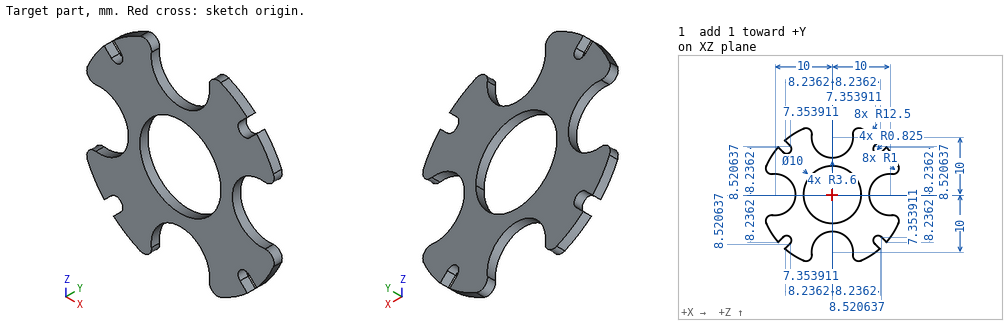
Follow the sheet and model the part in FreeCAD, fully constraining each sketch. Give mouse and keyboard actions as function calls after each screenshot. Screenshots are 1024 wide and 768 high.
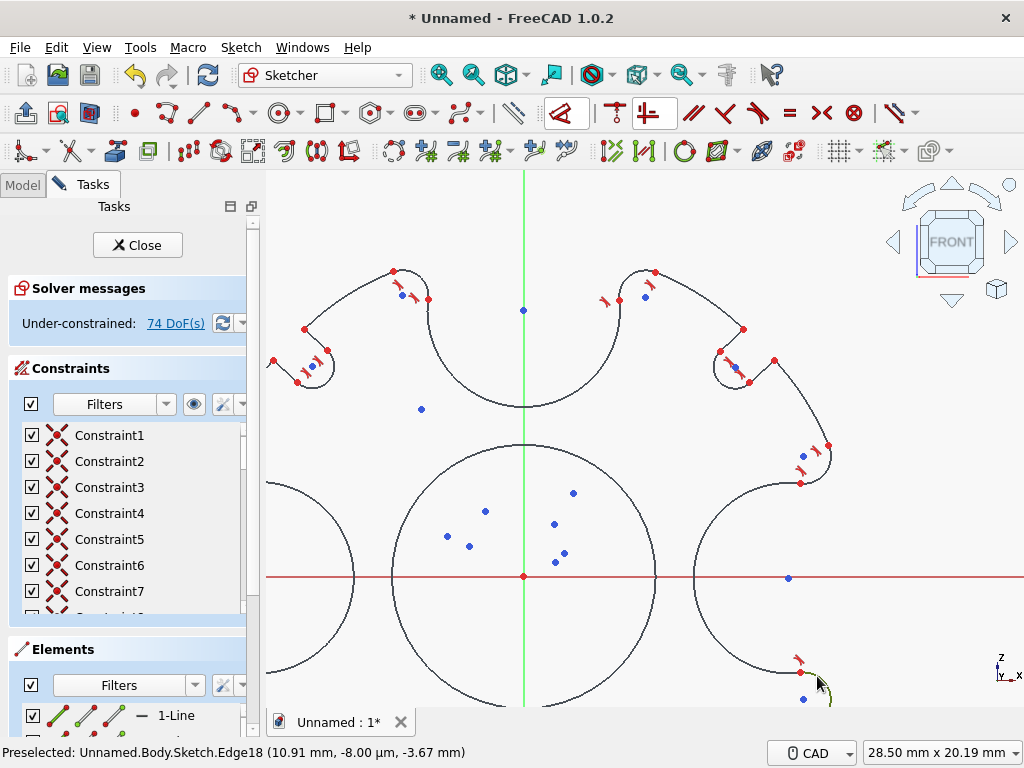
scroll(641, 270, down, 3)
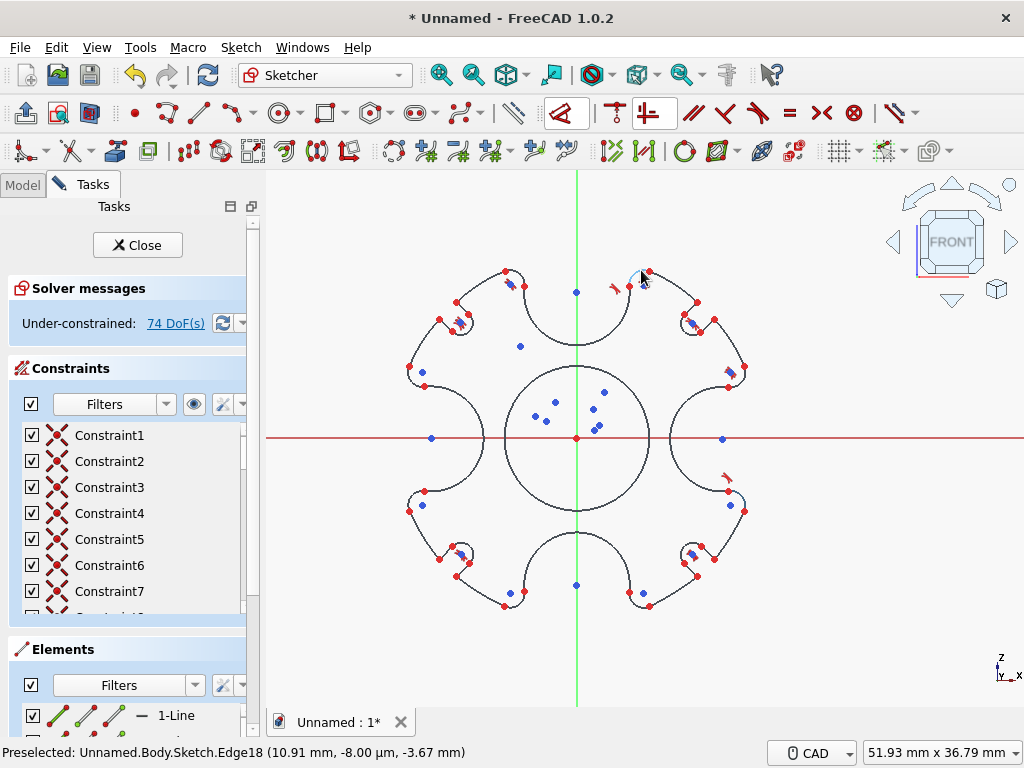
click(725, 546)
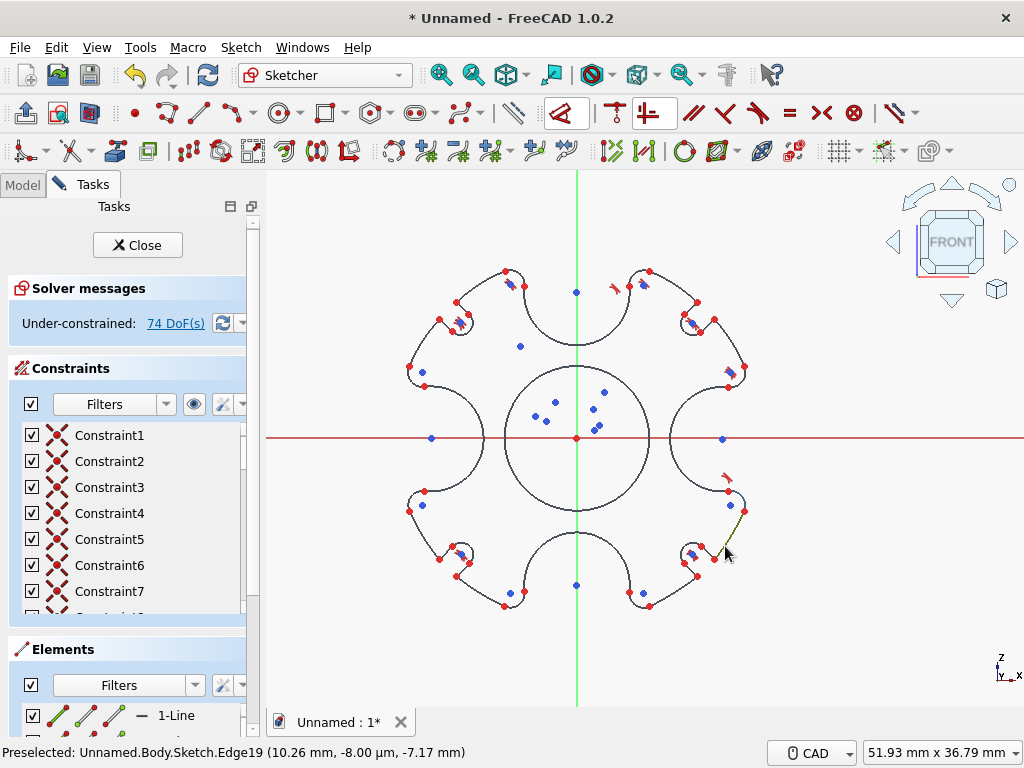
click(758, 114)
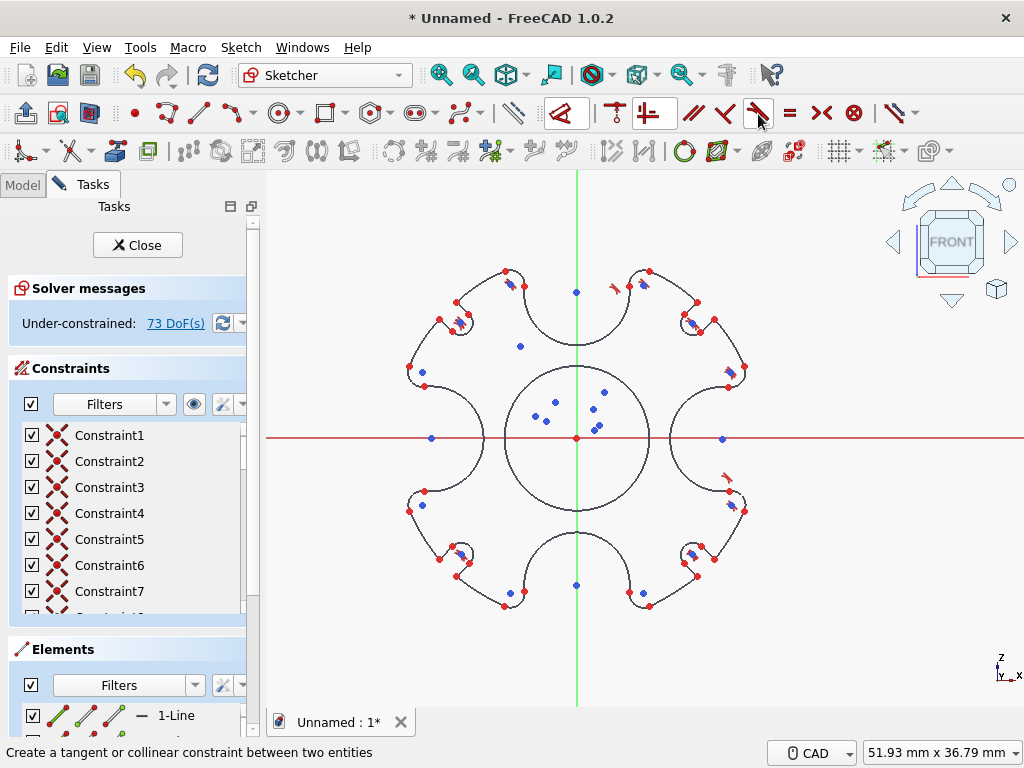
click(665, 599)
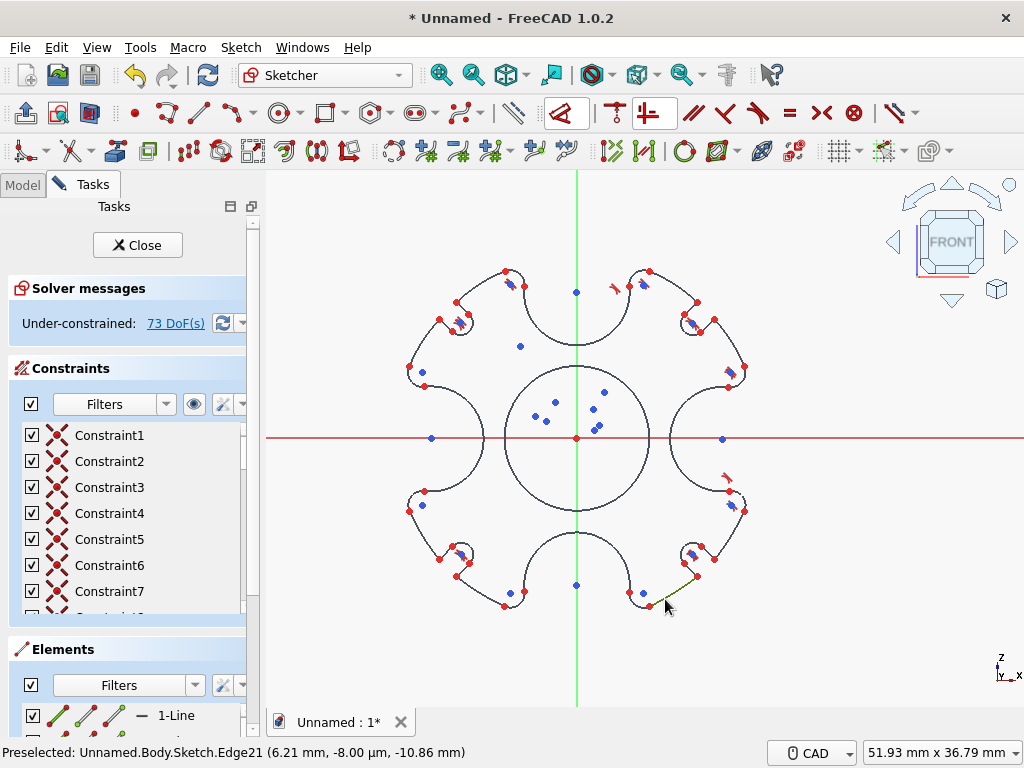
click(635, 605)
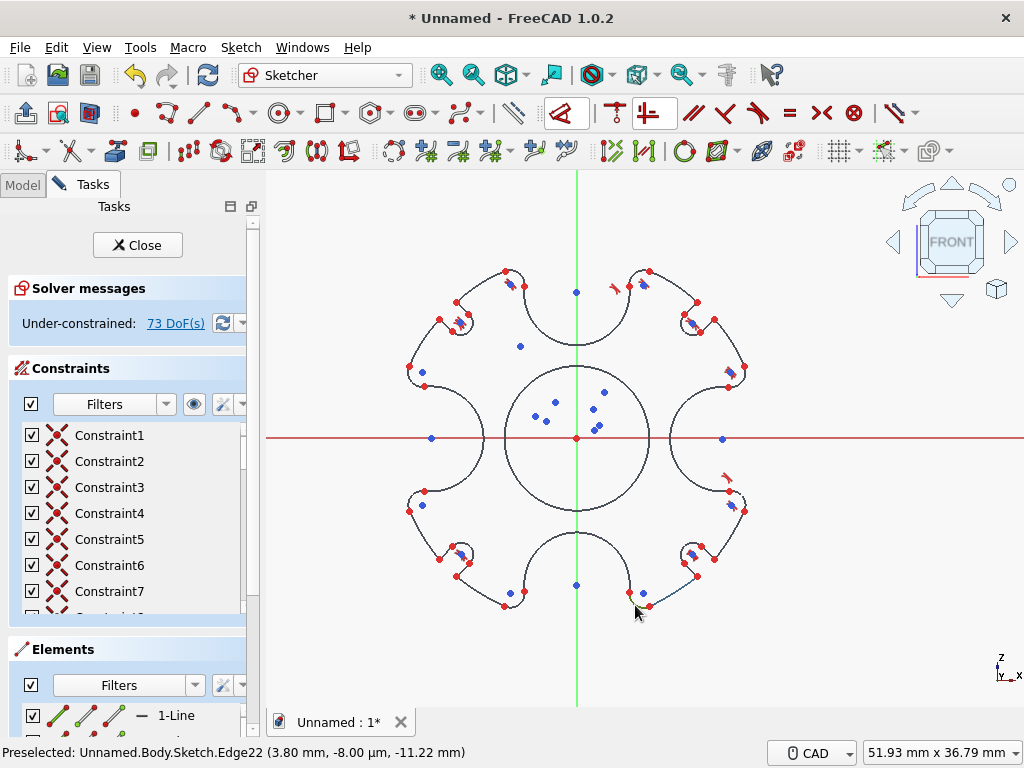
click(758, 114)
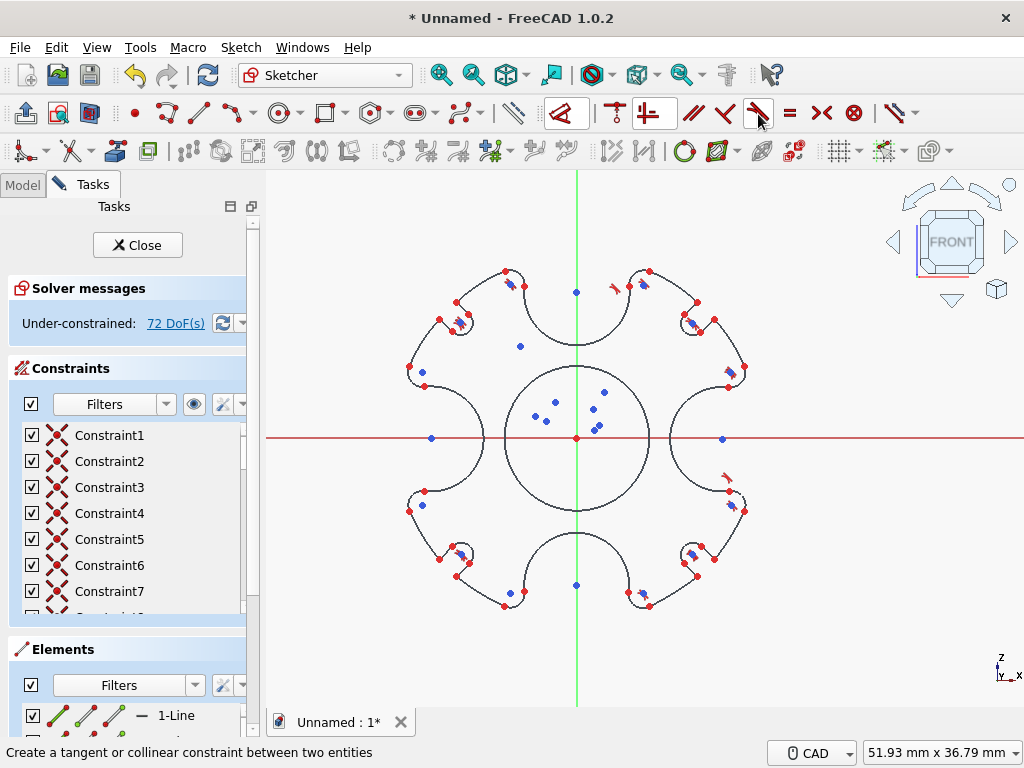
scroll(631, 601, up, 3)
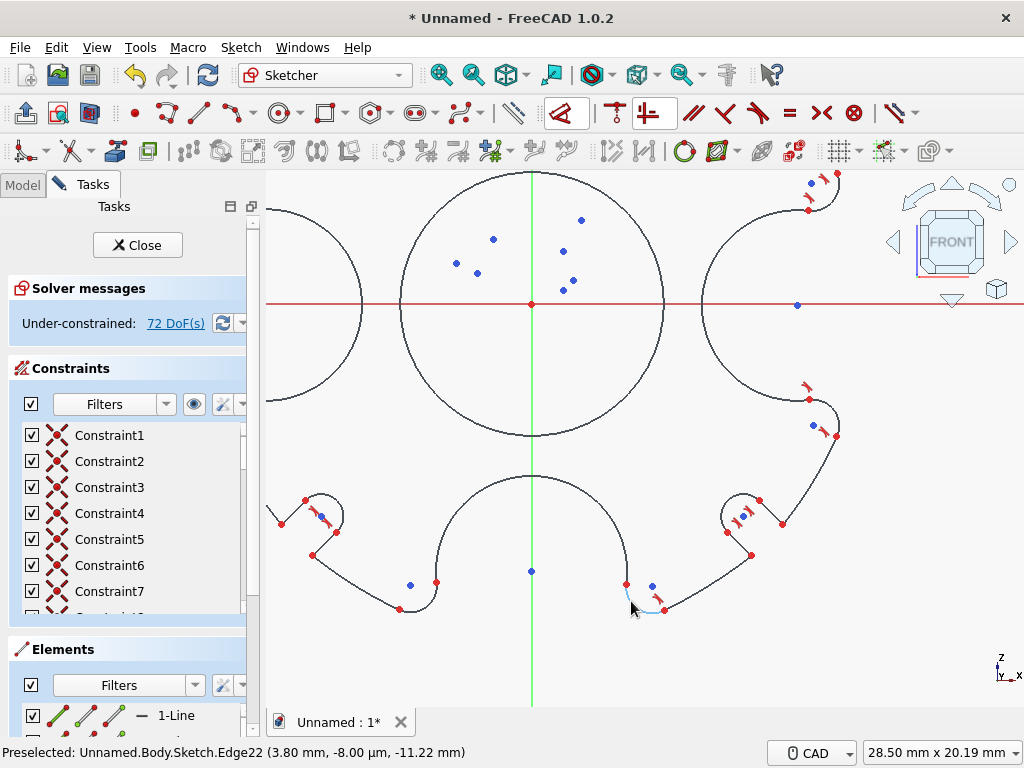
click(630, 601)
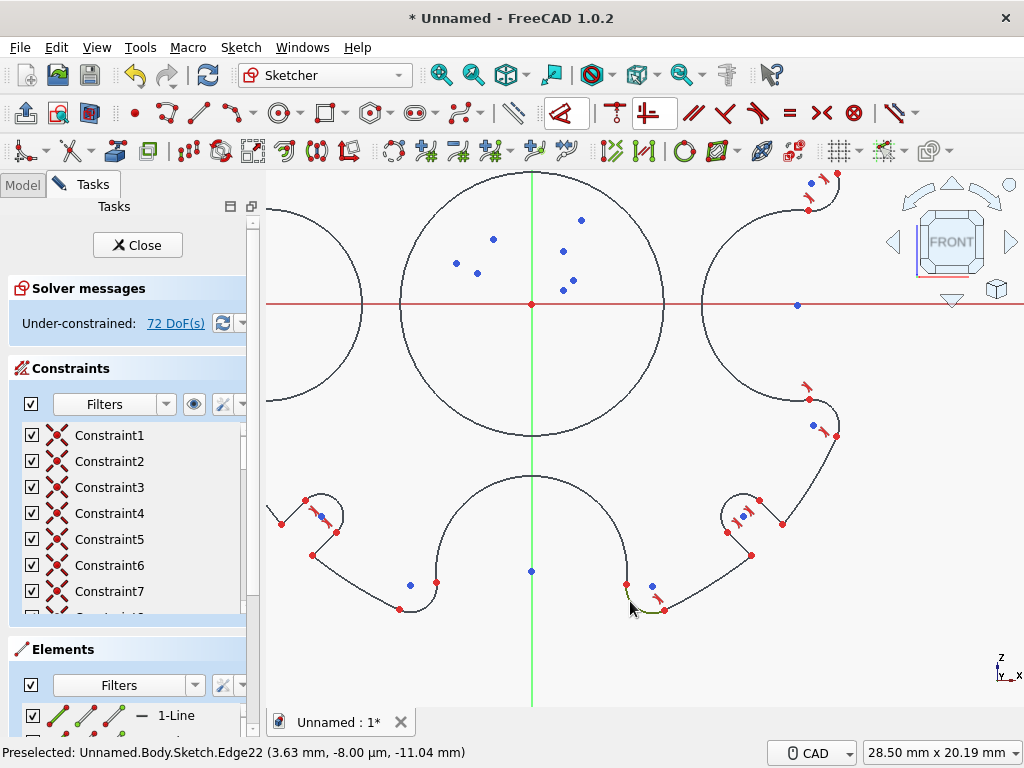
click(592, 498)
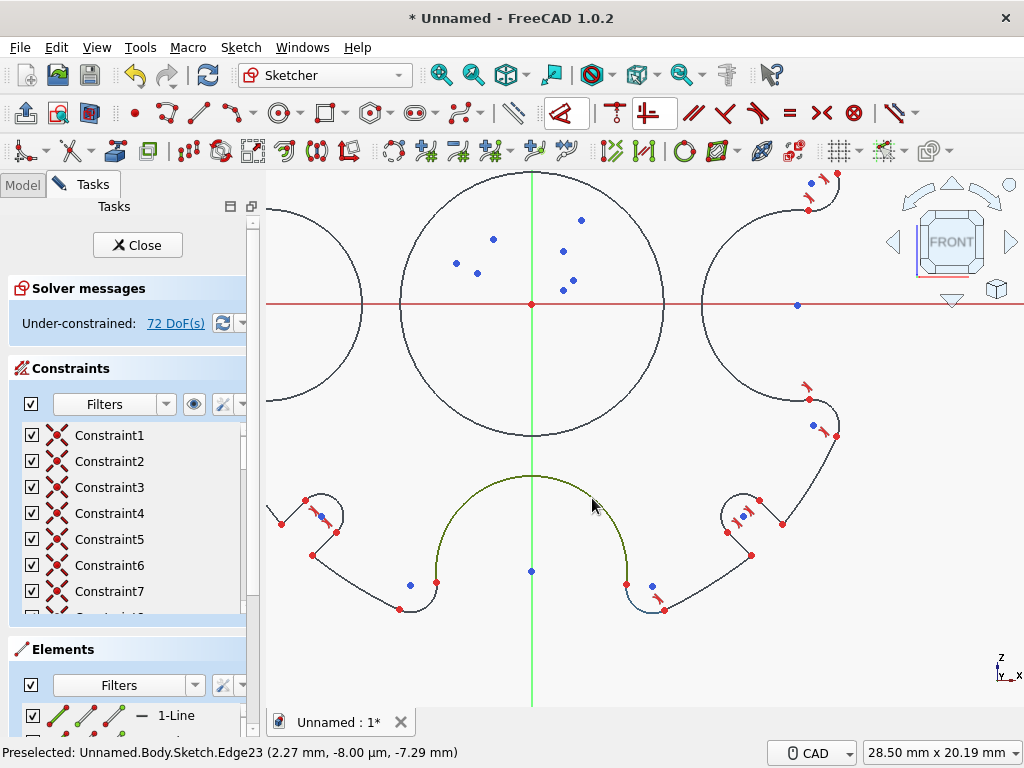
click(758, 114)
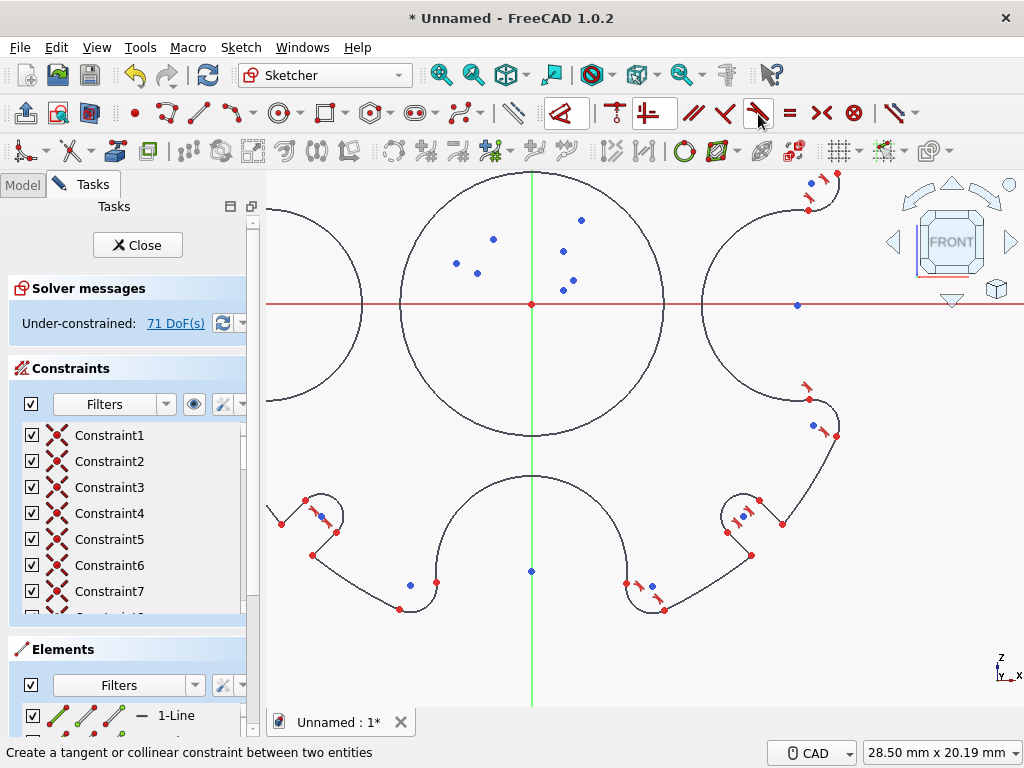
click(592, 497)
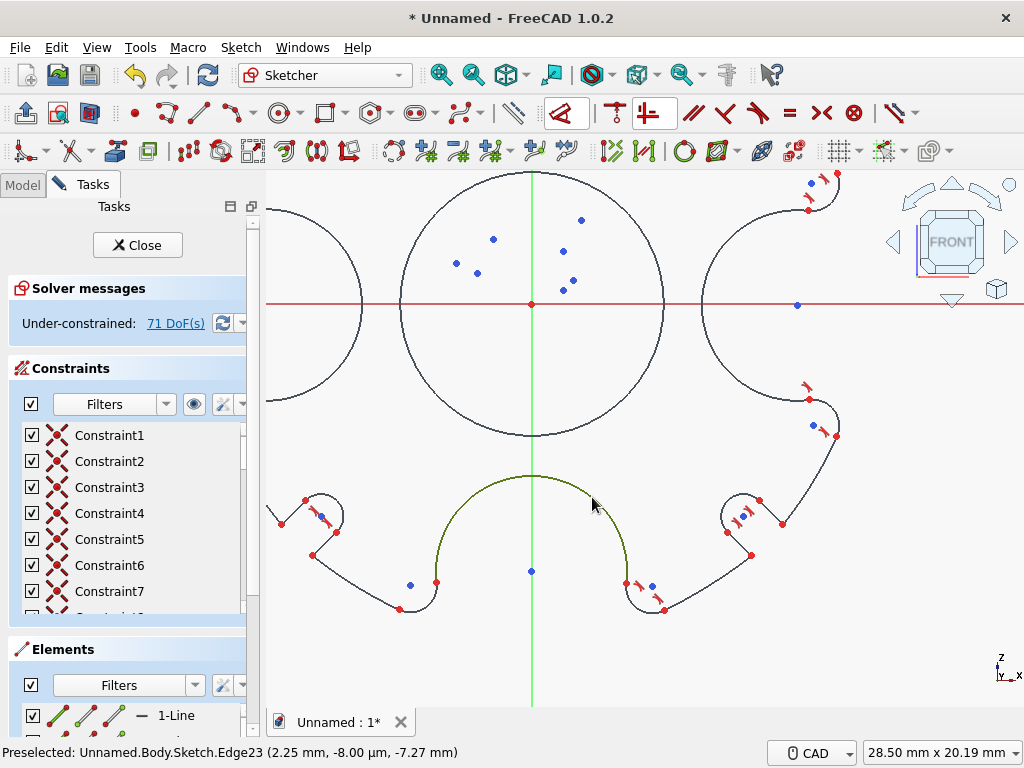
click(416, 612)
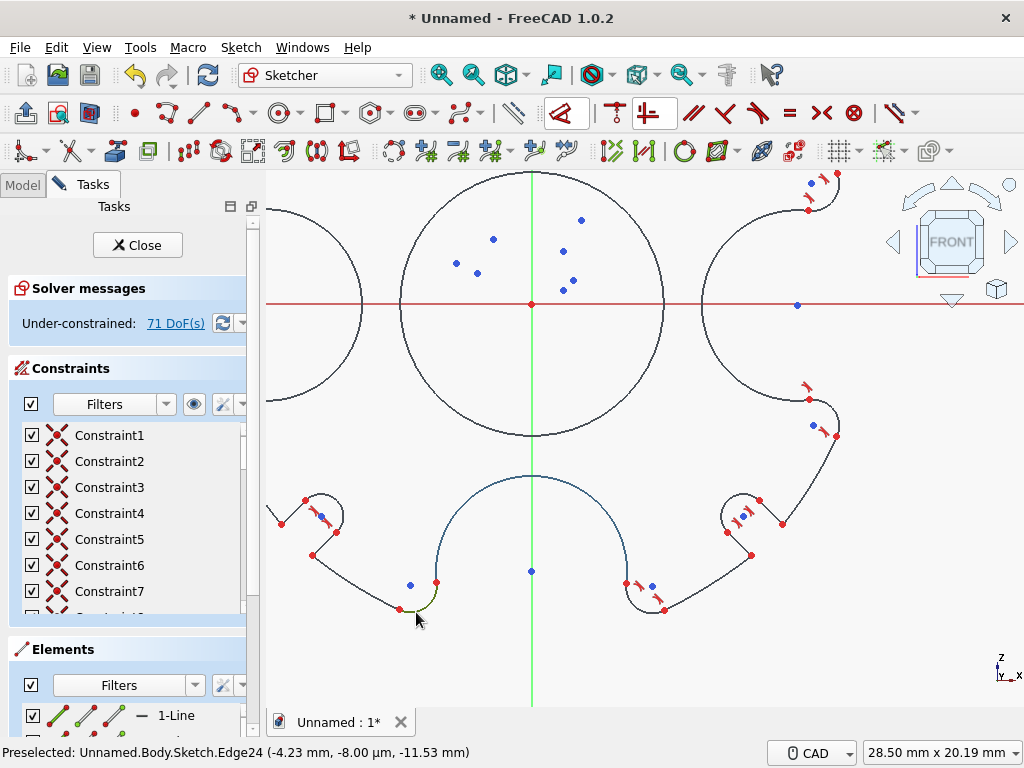
click(758, 114)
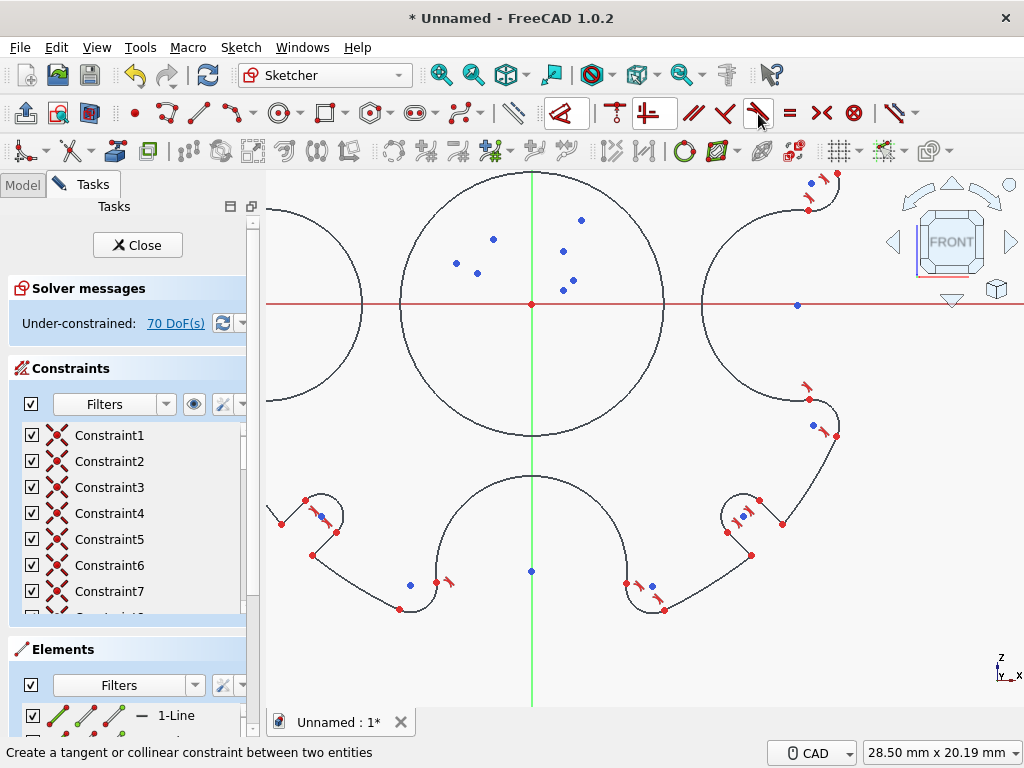
click(416, 612)